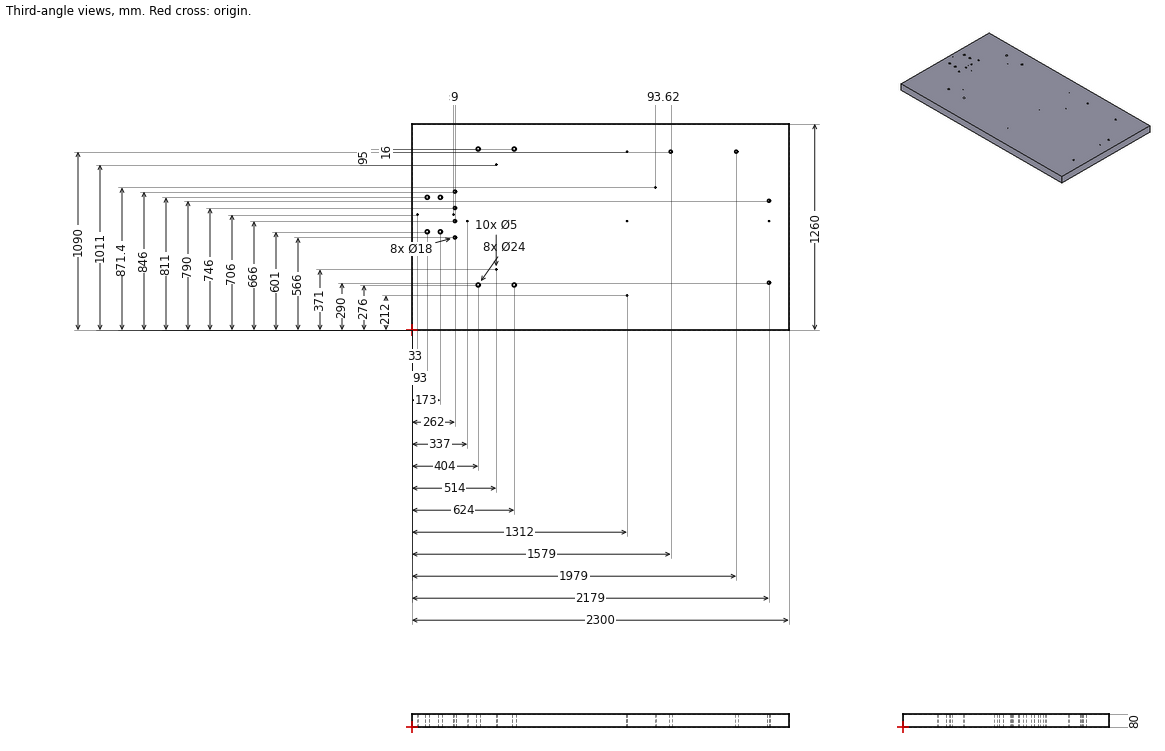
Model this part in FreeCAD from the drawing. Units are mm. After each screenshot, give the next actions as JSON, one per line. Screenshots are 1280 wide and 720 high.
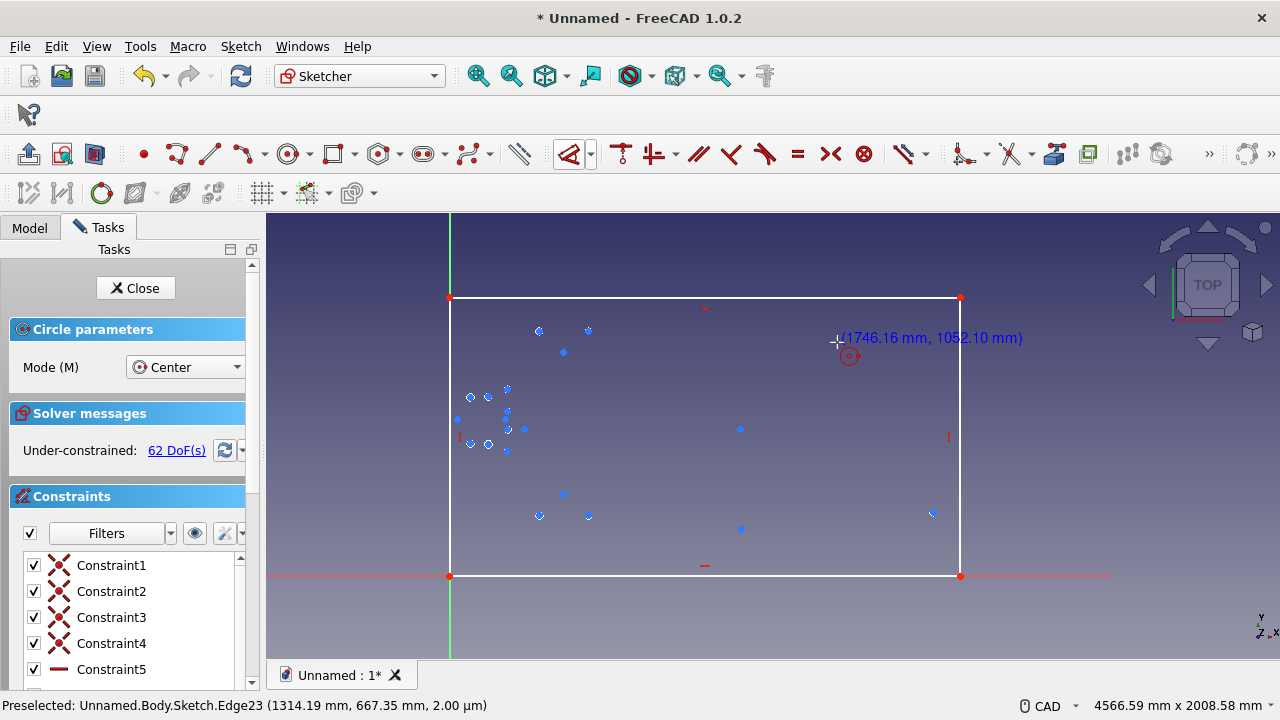
{"action": "left_click", "coordinate": [779, 383]}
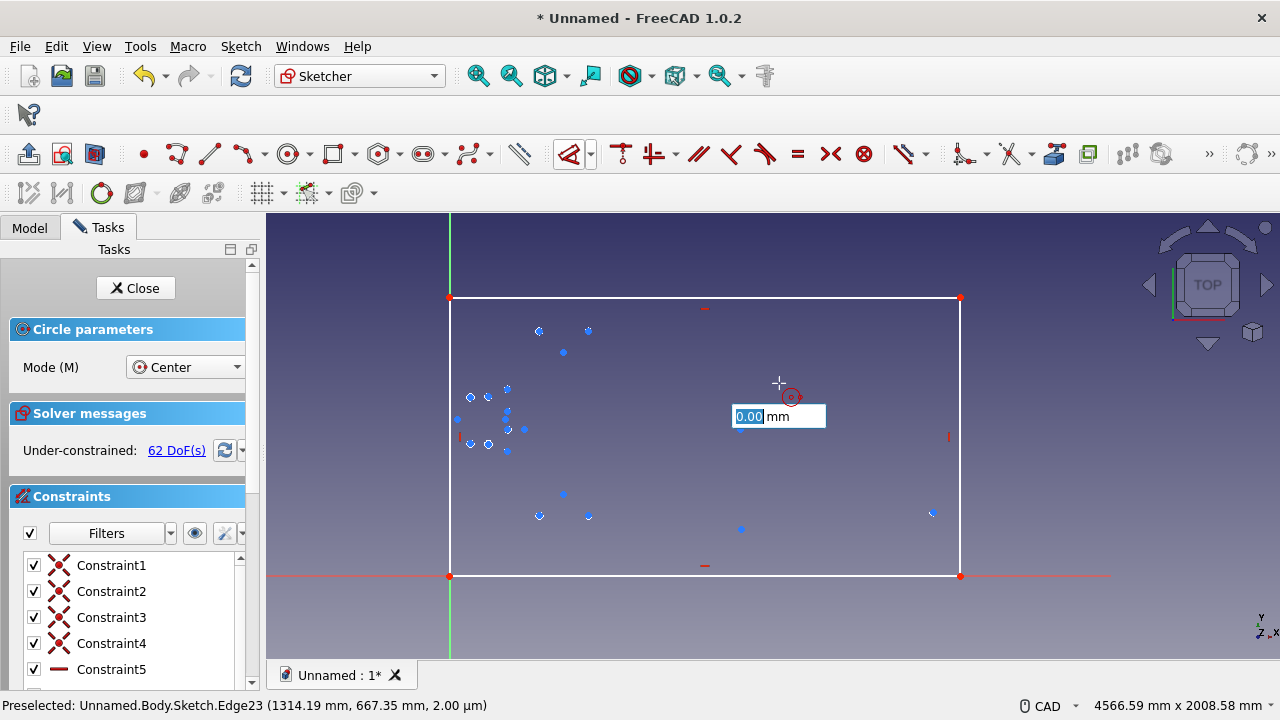
{"action": "scroll", "coordinate": [780, 382], "scroll_direction": "up", "scroll_amount": 17}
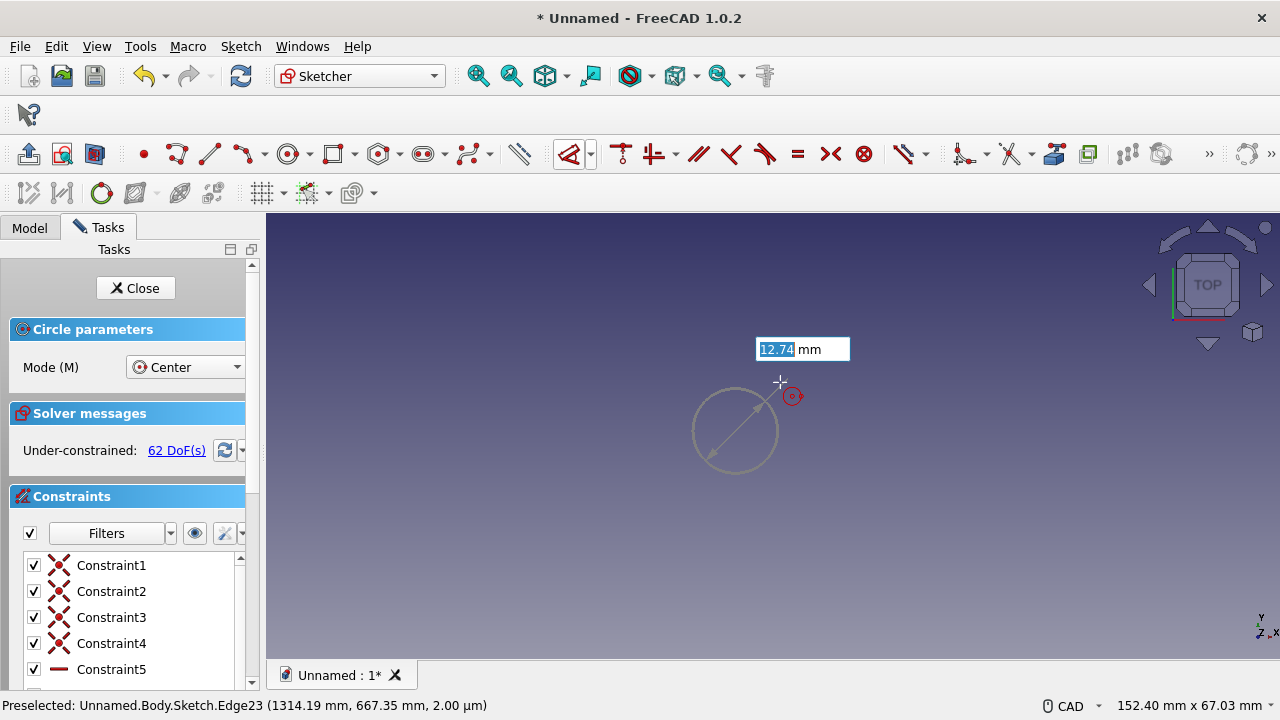
{"action": "left_click", "coordinate": [759, 381]}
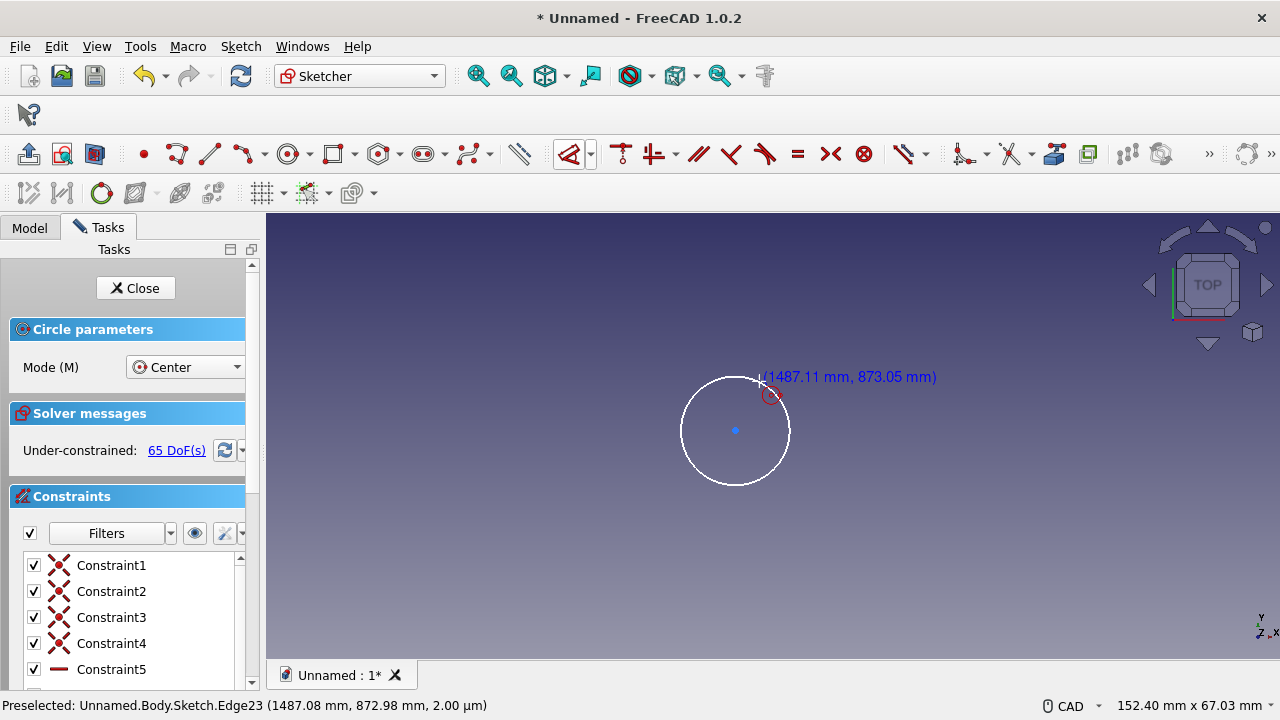
{"action": "scroll", "coordinate": [780, 382], "scroll_direction": "down", "scroll_amount": 17}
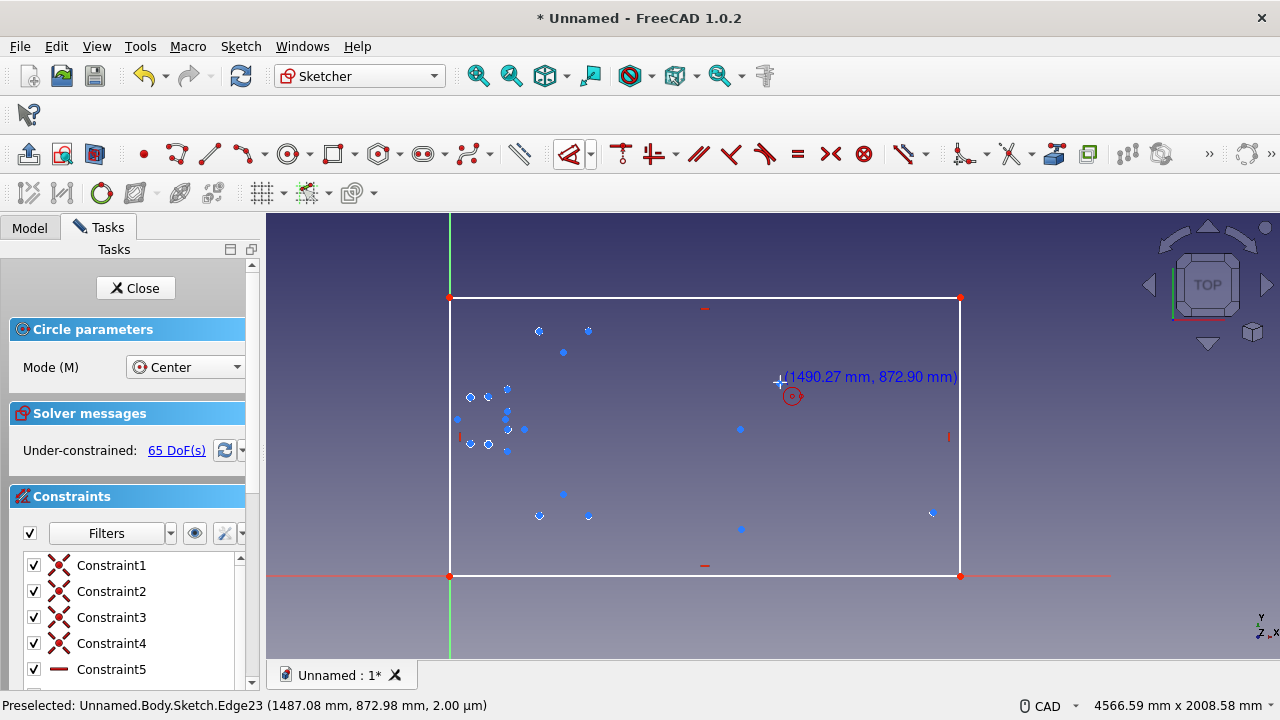
{"action": "scroll", "coordinate": [933, 428], "scroll_direction": "up", "scroll_amount": 19}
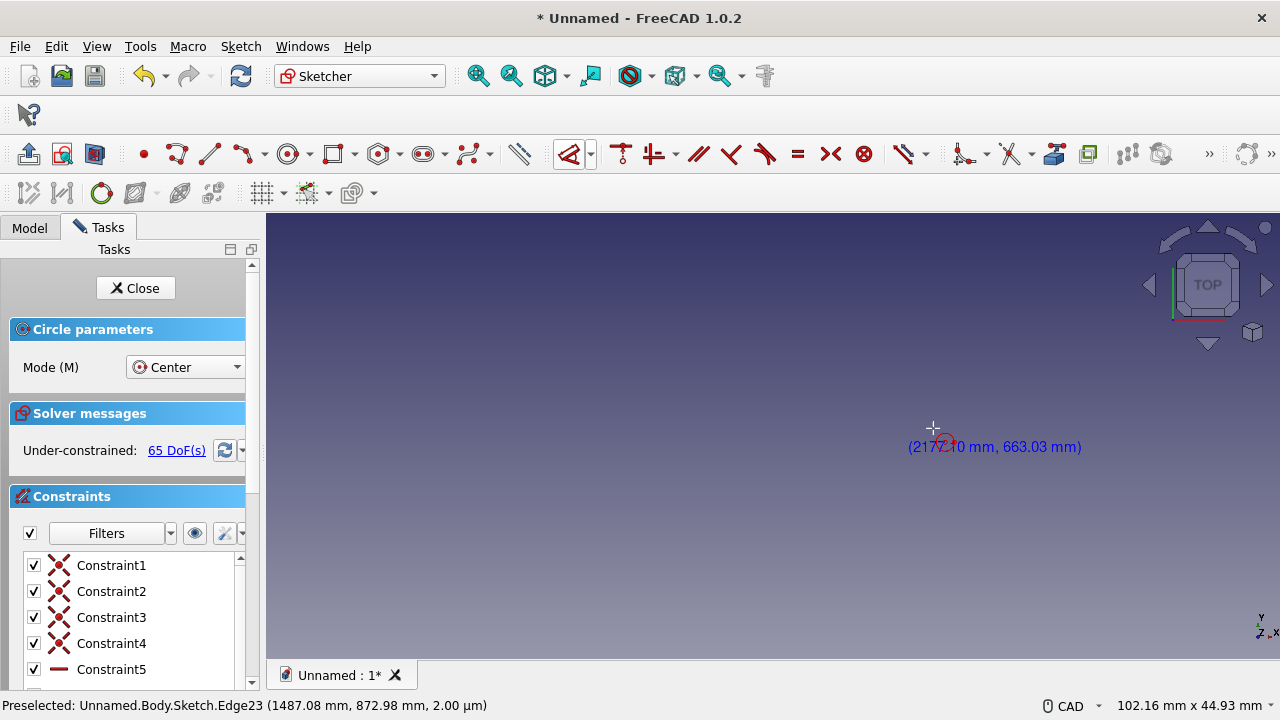
{"action": "scroll", "coordinate": [704, 436], "scroll_direction": "down", "scroll_amount": 15}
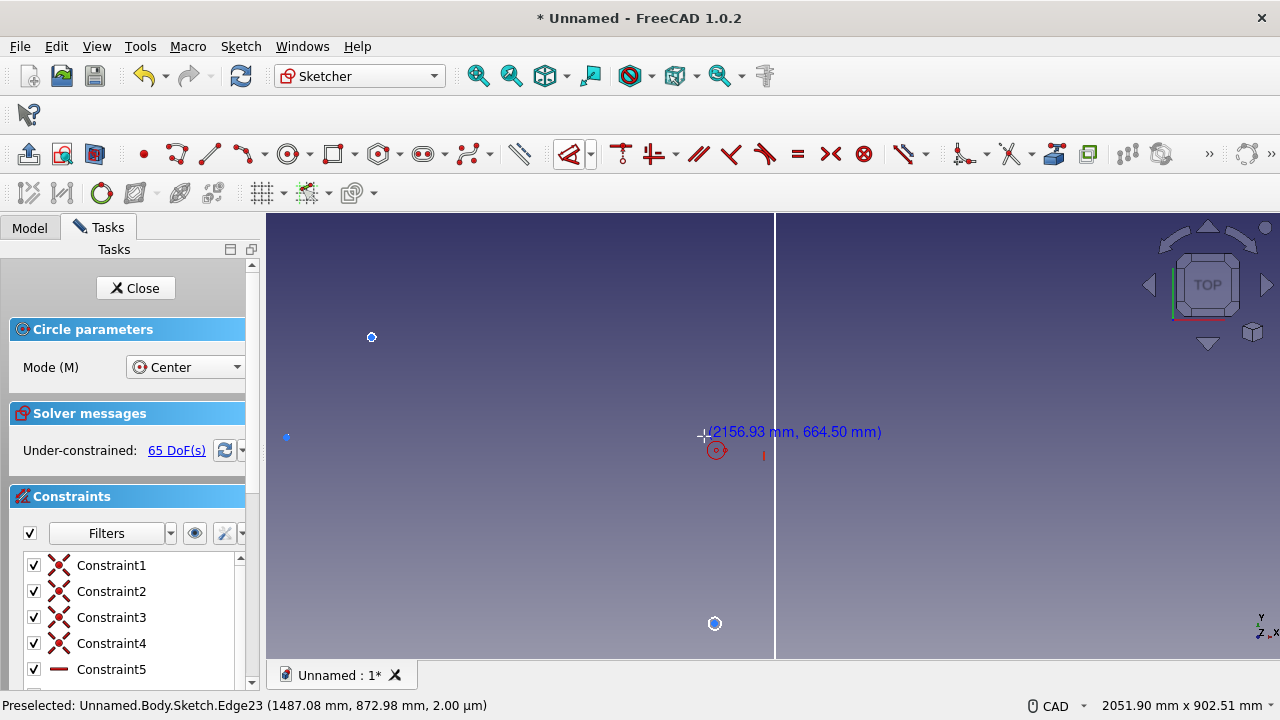
{"action": "scroll", "coordinate": [1111, 422], "scroll_direction": "down", "scroll_amount": 4}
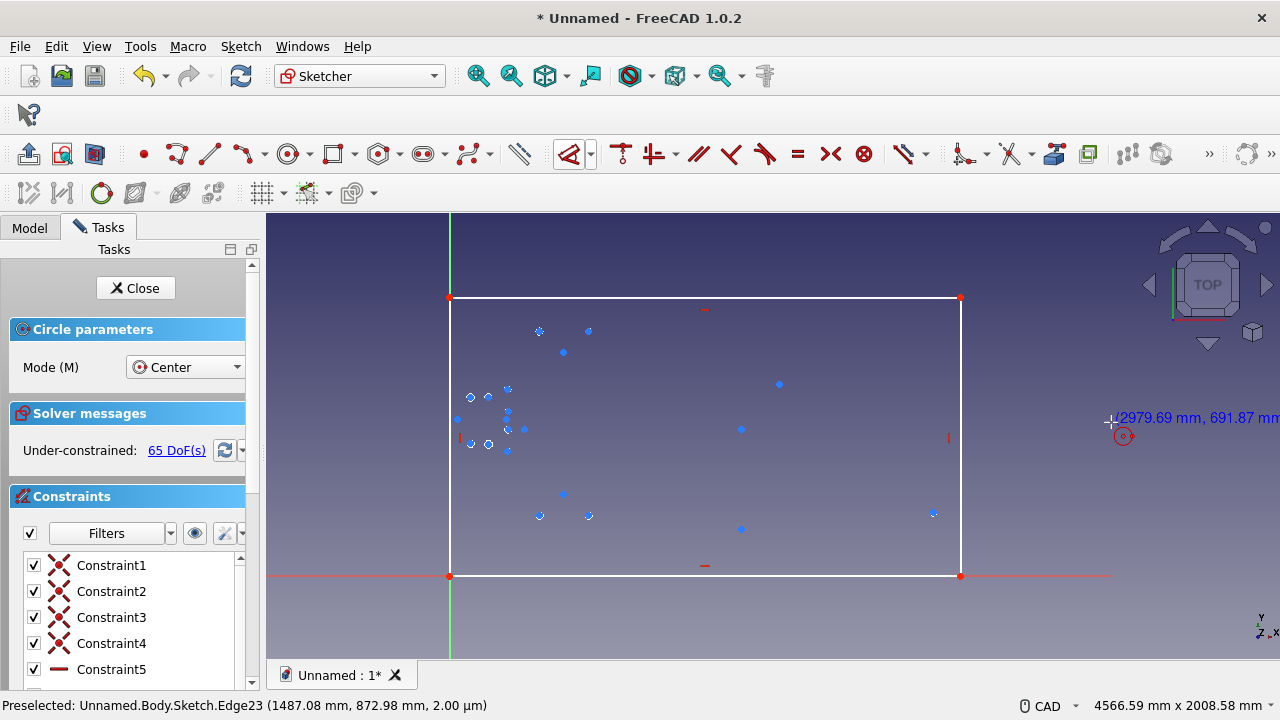
{"action": "left_click", "coordinate": [934, 428]}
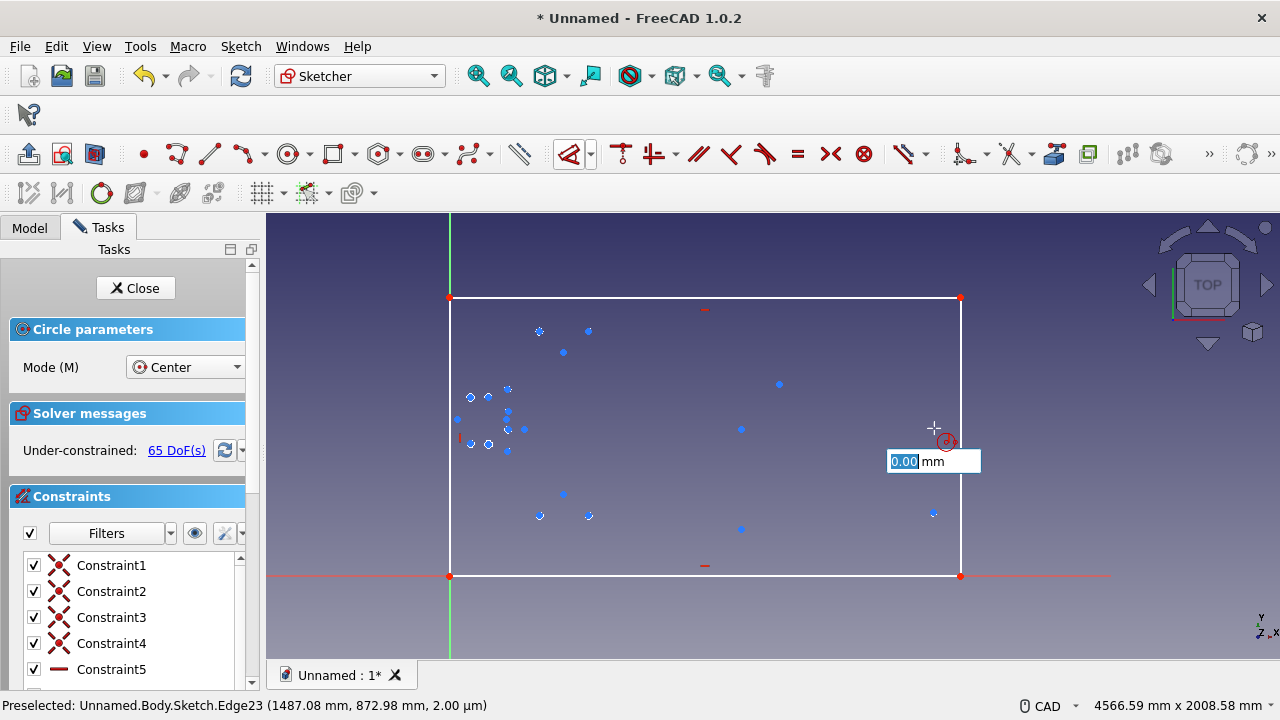
{"action": "scroll", "coordinate": [934, 428], "scroll_direction": "up", "scroll_amount": 17}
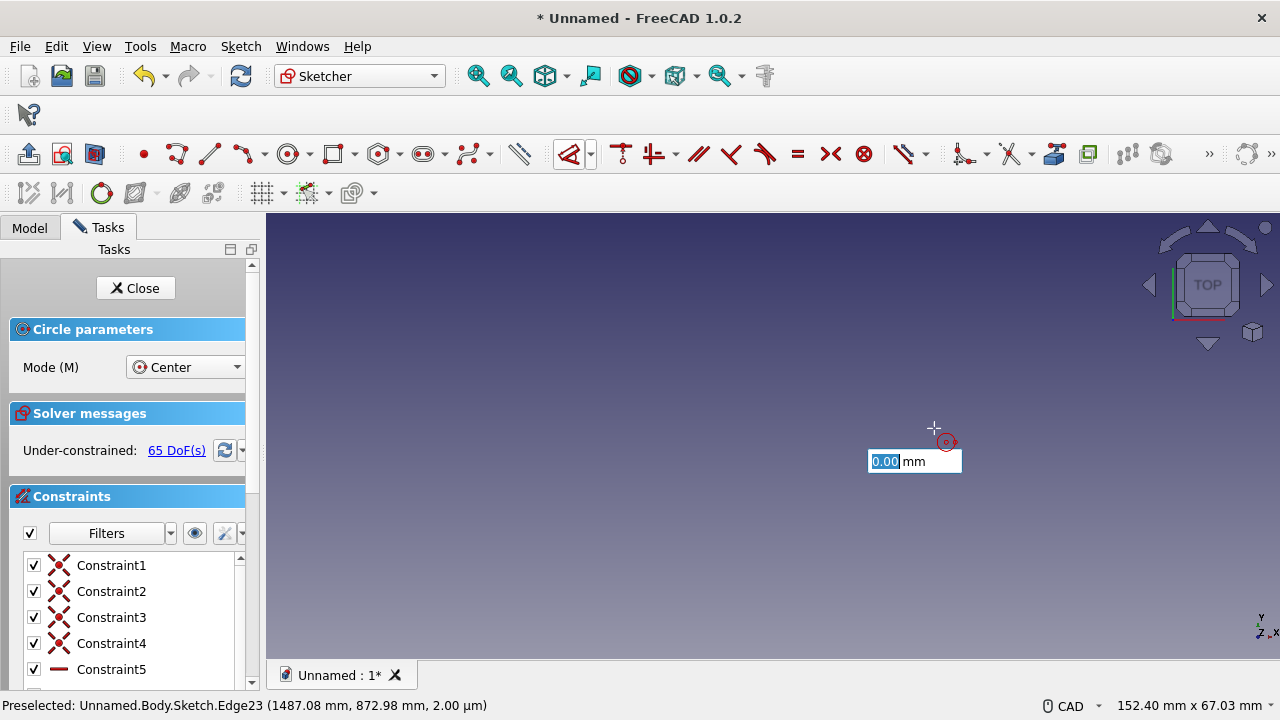
{"action": "left_click", "coordinate": [917, 416]}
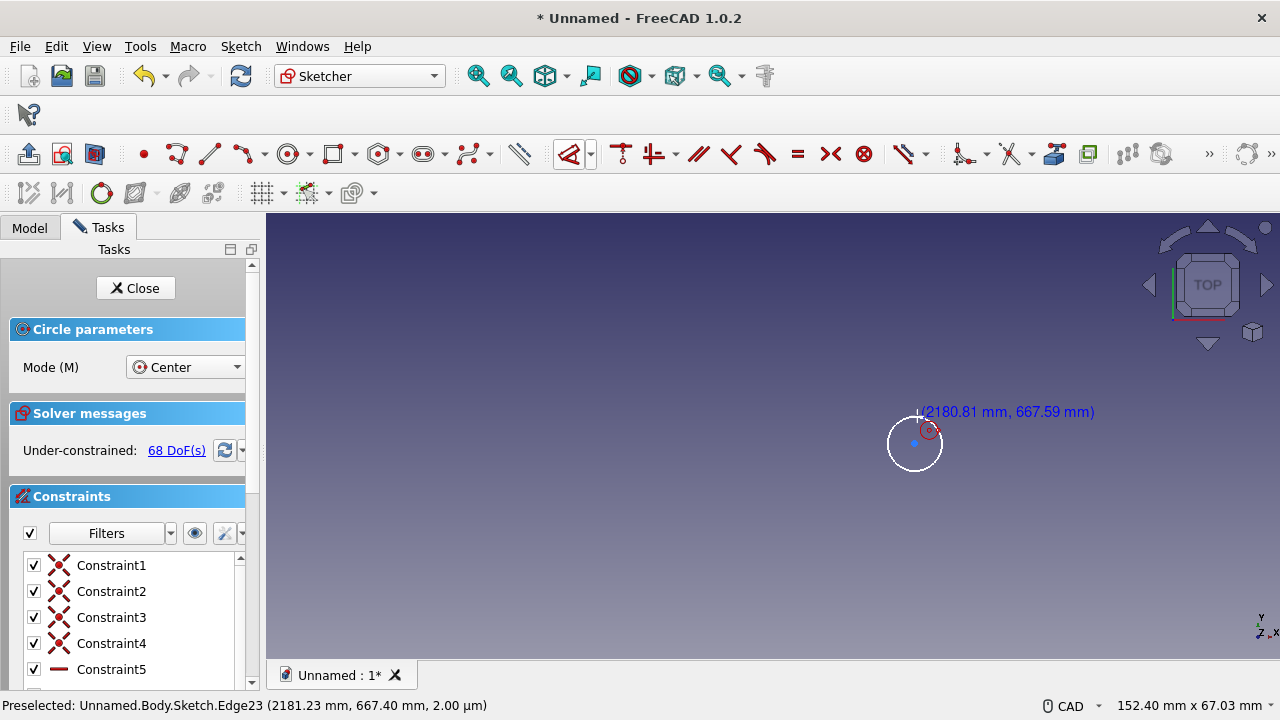
{"action": "scroll", "coordinate": [934, 428], "scroll_direction": "down", "scroll_amount": 17}